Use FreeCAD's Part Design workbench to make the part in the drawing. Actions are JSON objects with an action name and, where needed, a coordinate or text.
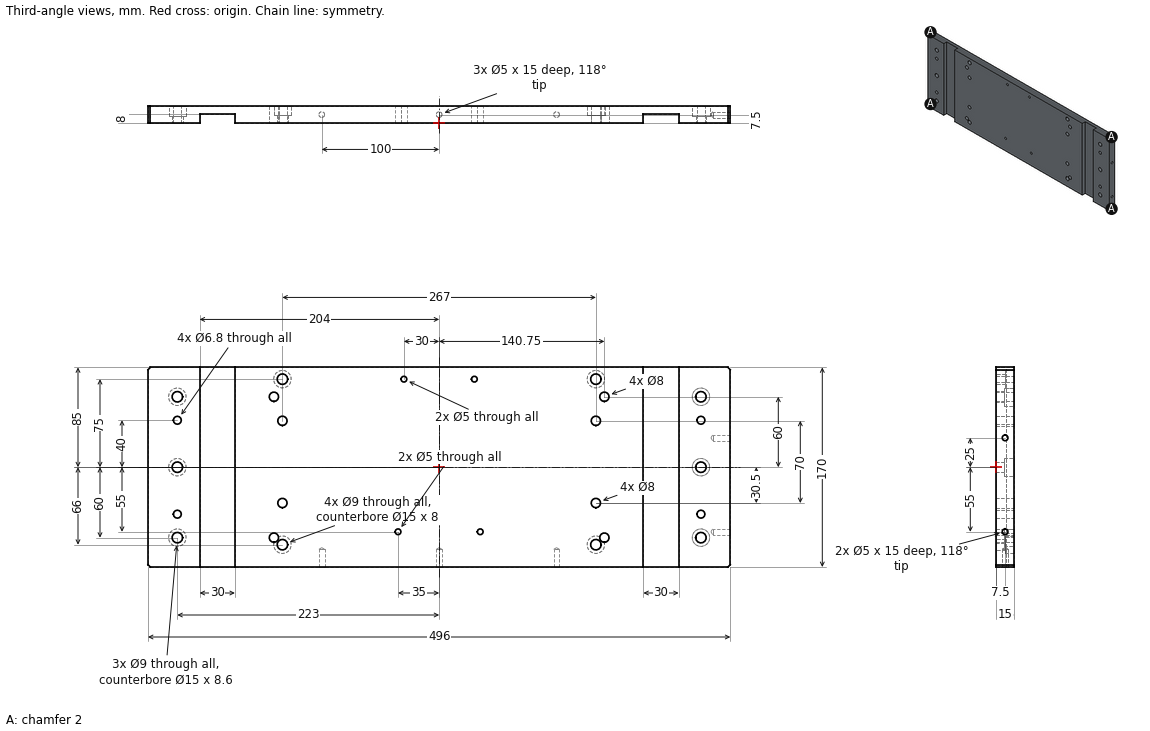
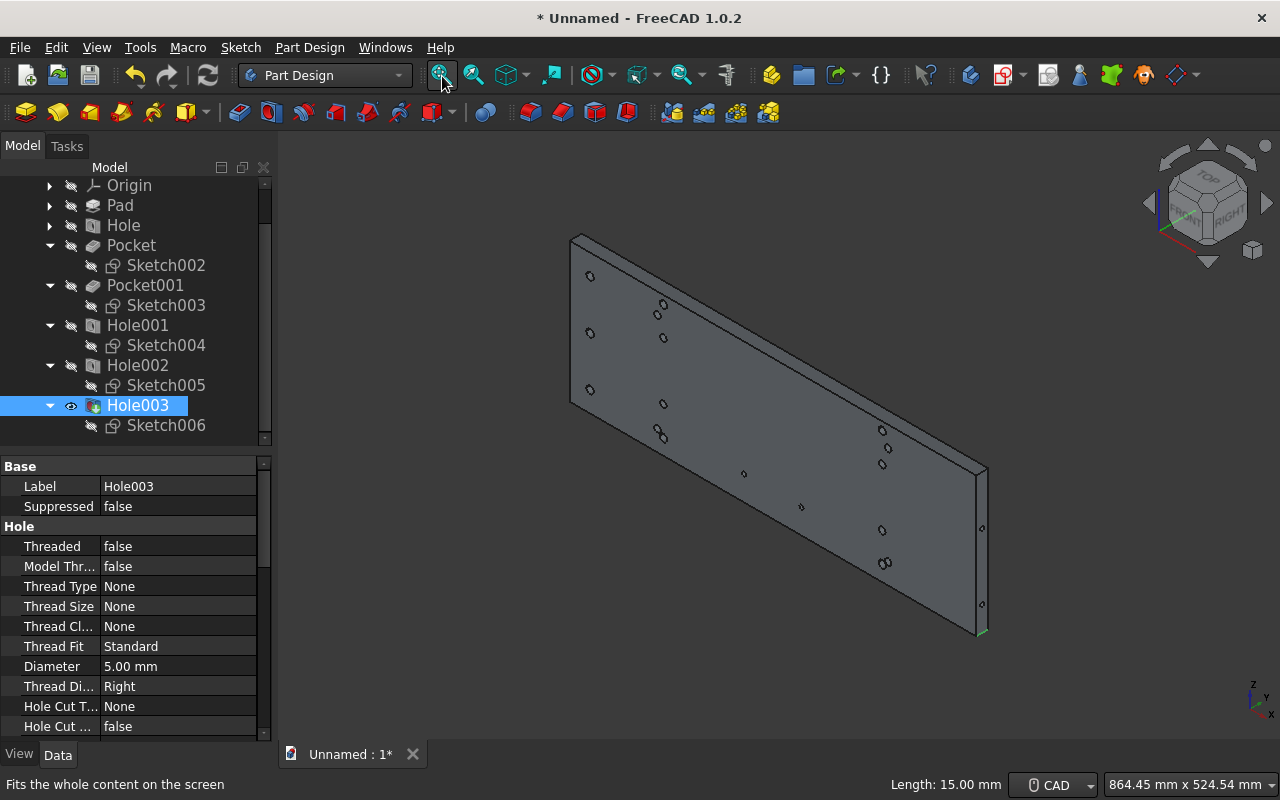
{"action": "left_click", "coordinate": [982, 471], "text": "ctrl"}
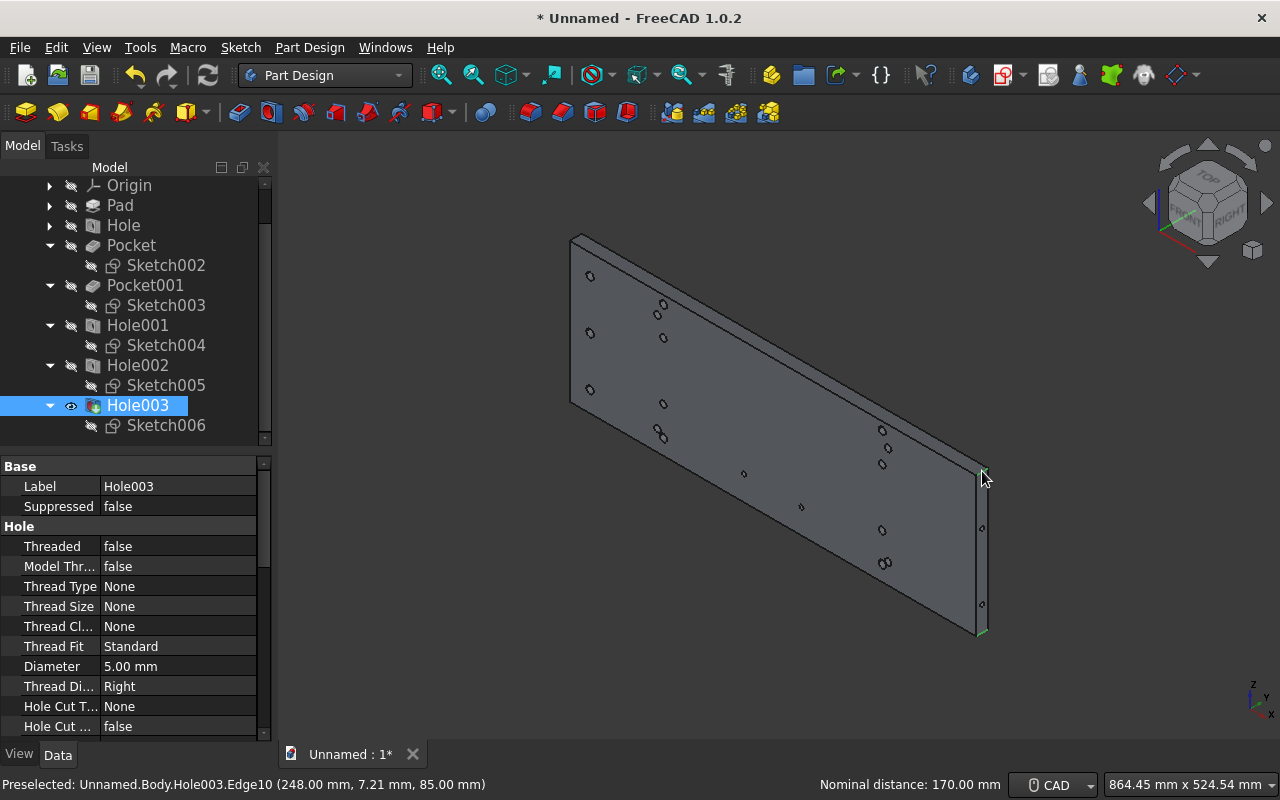
{"action": "scroll", "coordinate": [576, 236], "scroll_direction": "up", "scroll_amount": 5}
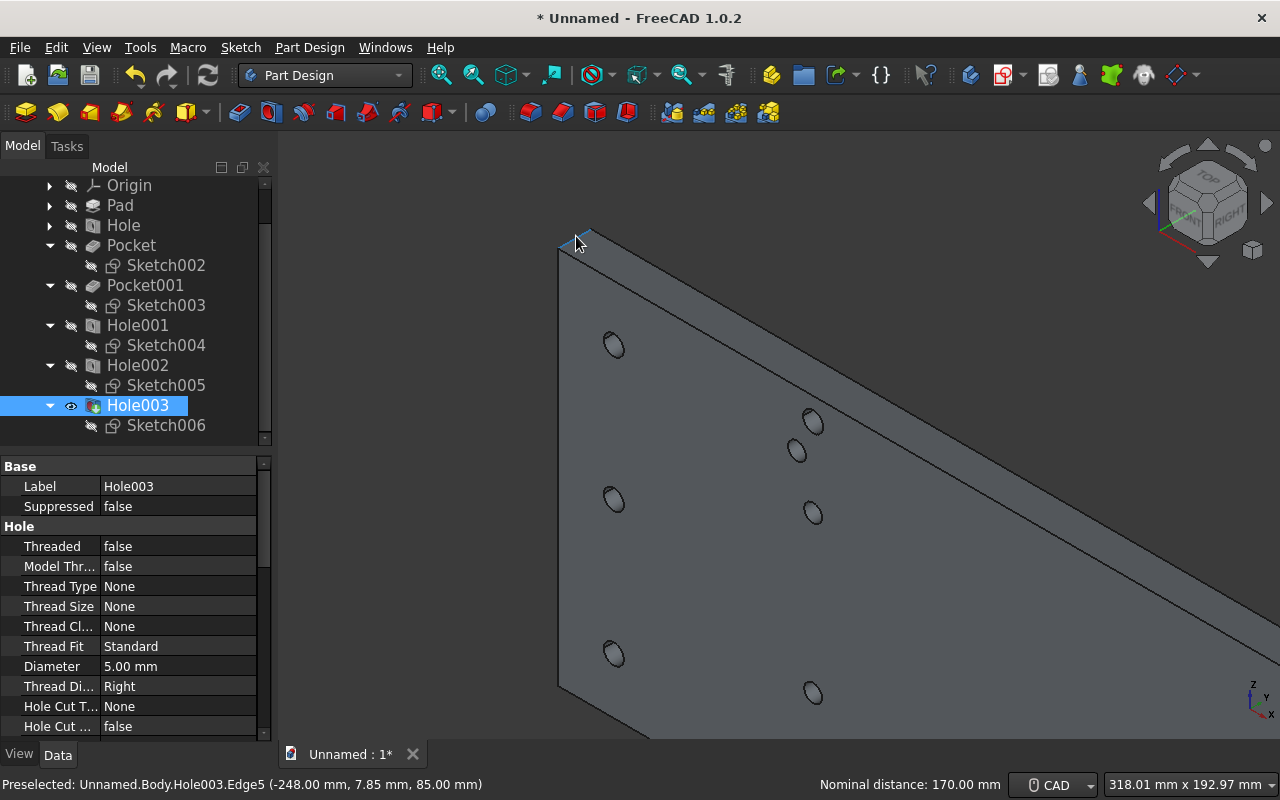
{"action": "left_click", "coordinate": [442, 76]}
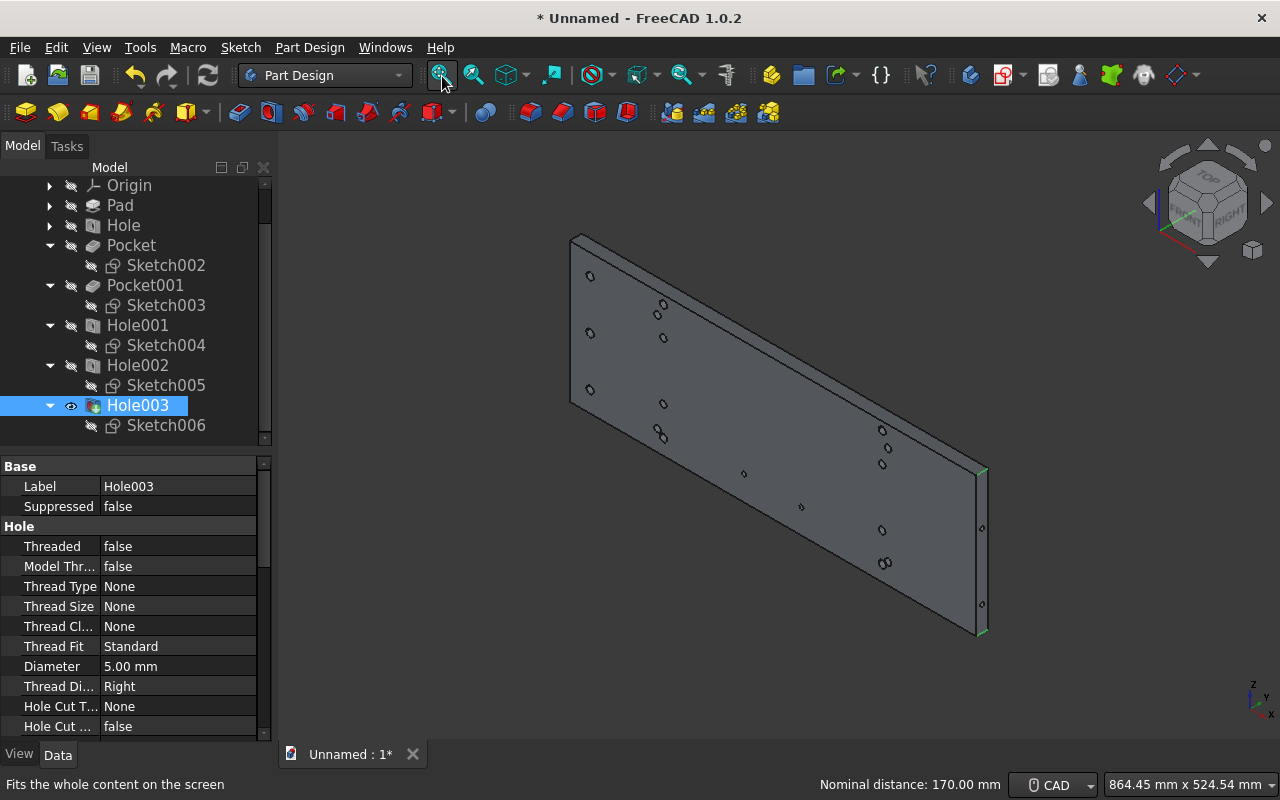
{"action": "key", "text": "2"}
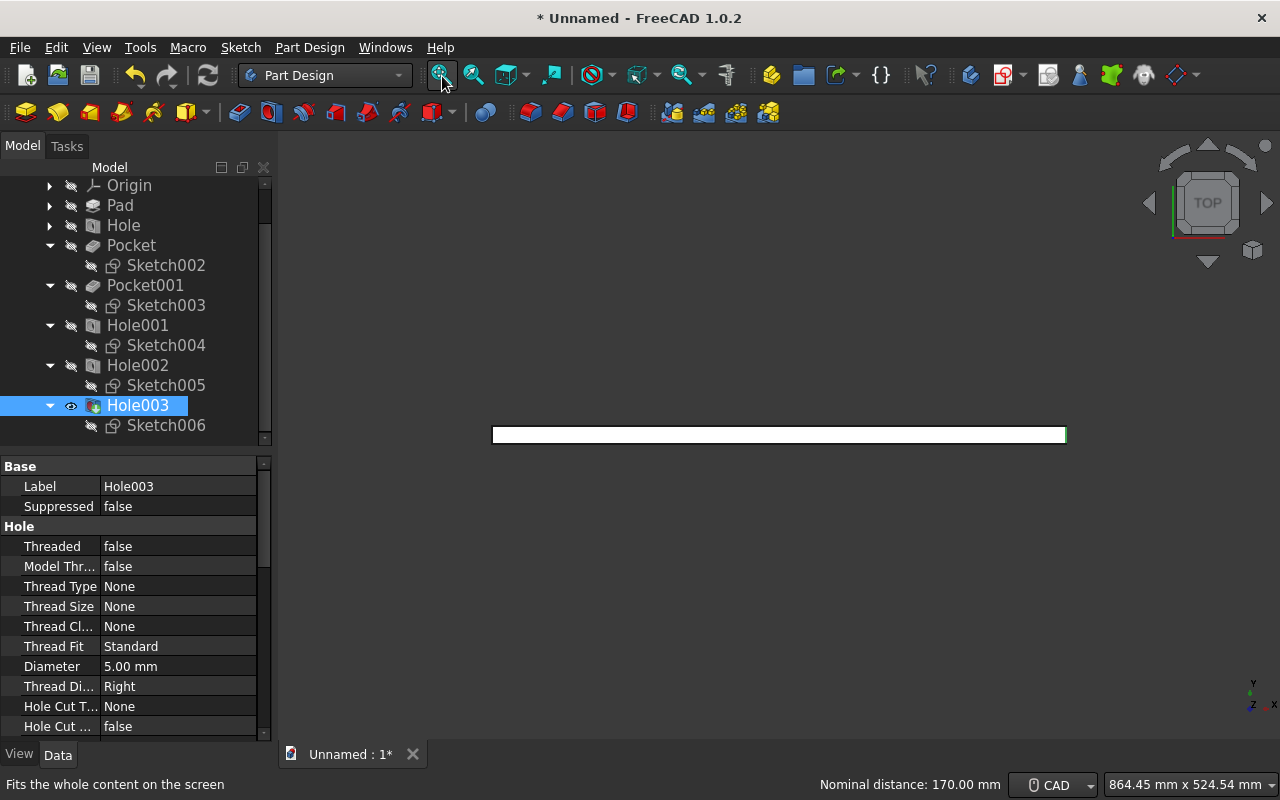
{"action": "left_click", "coordinate": [492, 434], "text": "ctrl"}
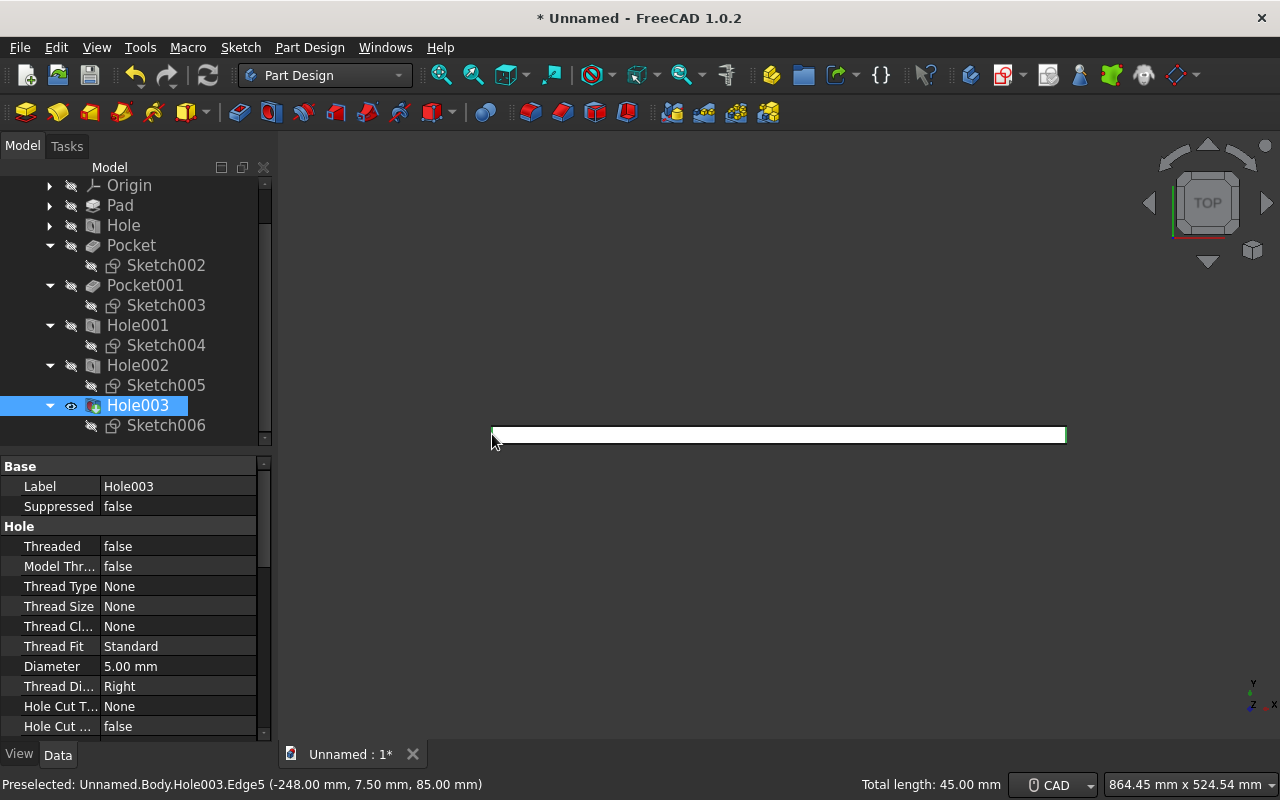
{"action": "scroll", "coordinate": [492, 434], "scroll_direction": "up", "scroll_amount": 5}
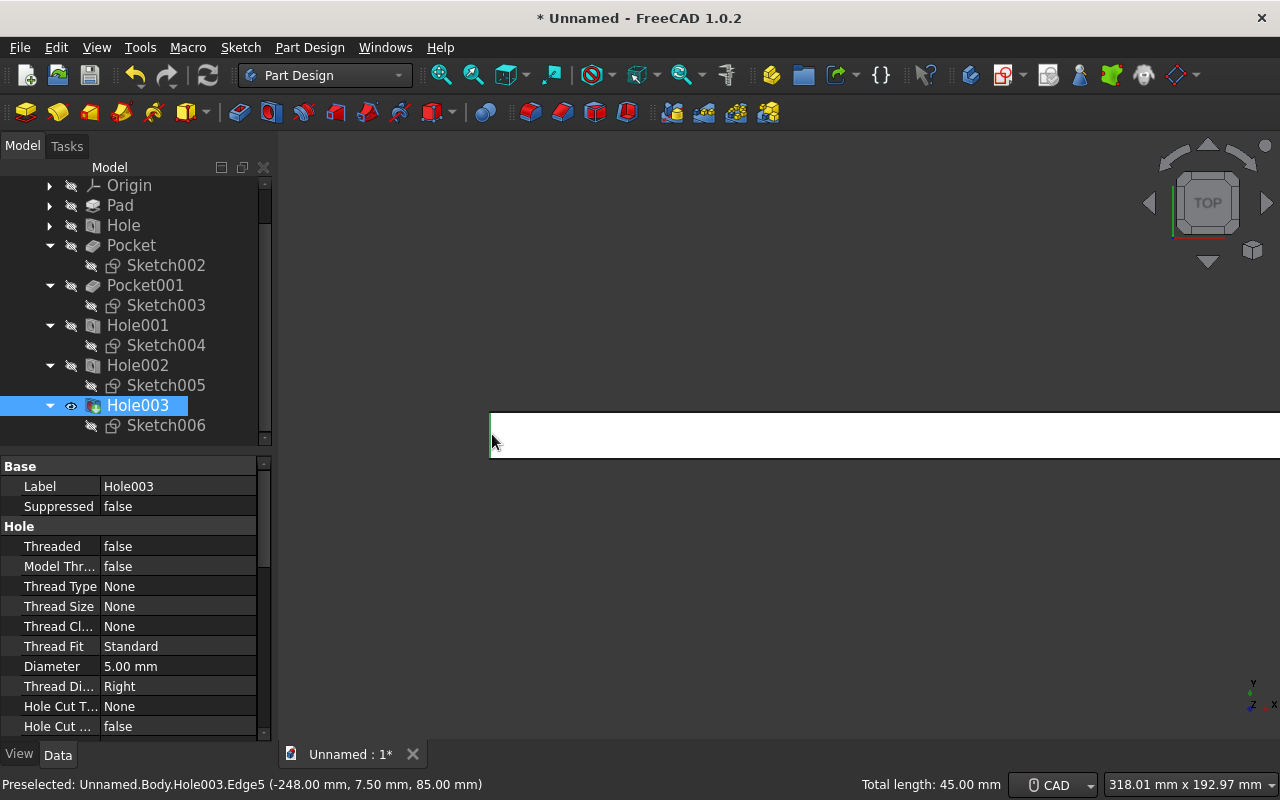
{"action": "left_click", "coordinate": [442, 76]}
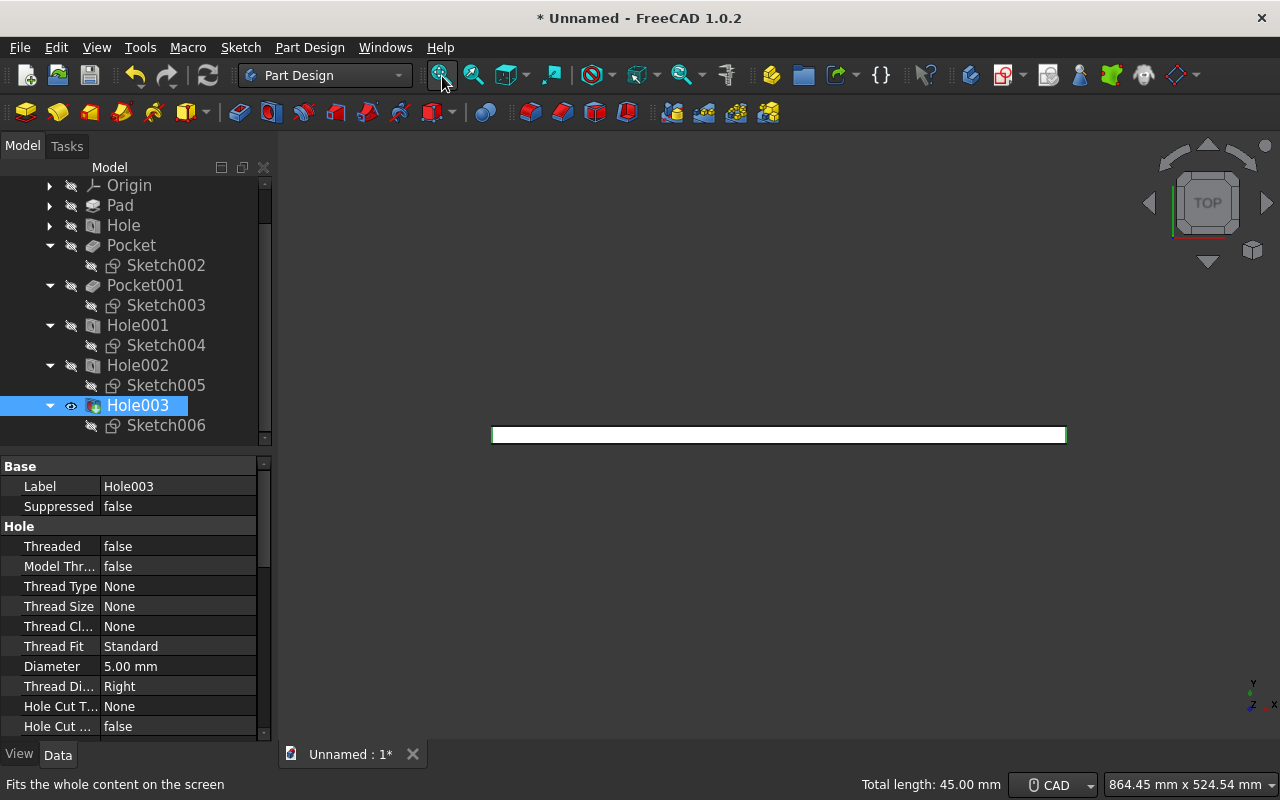
{"action": "key", "text": "1"}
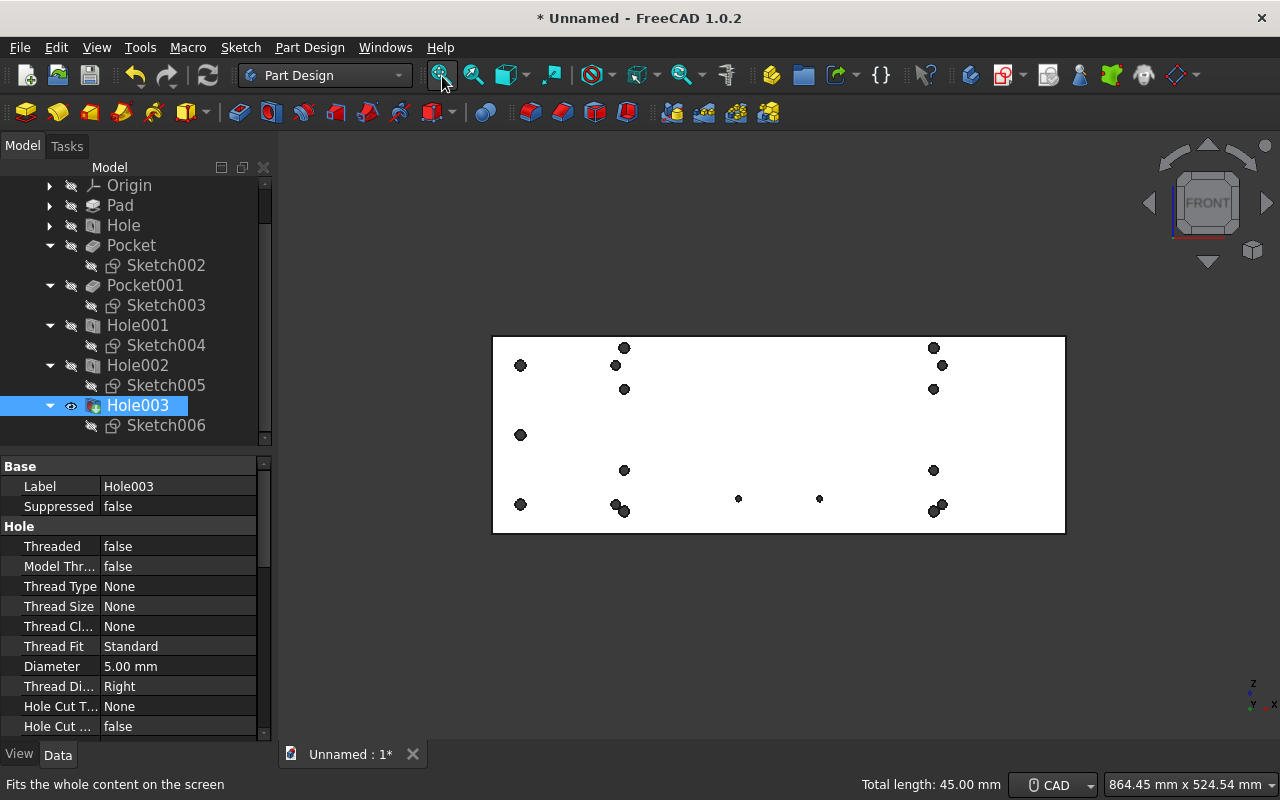
{"action": "scroll", "coordinate": [492, 533], "scroll_direction": "up", "scroll_amount": 5}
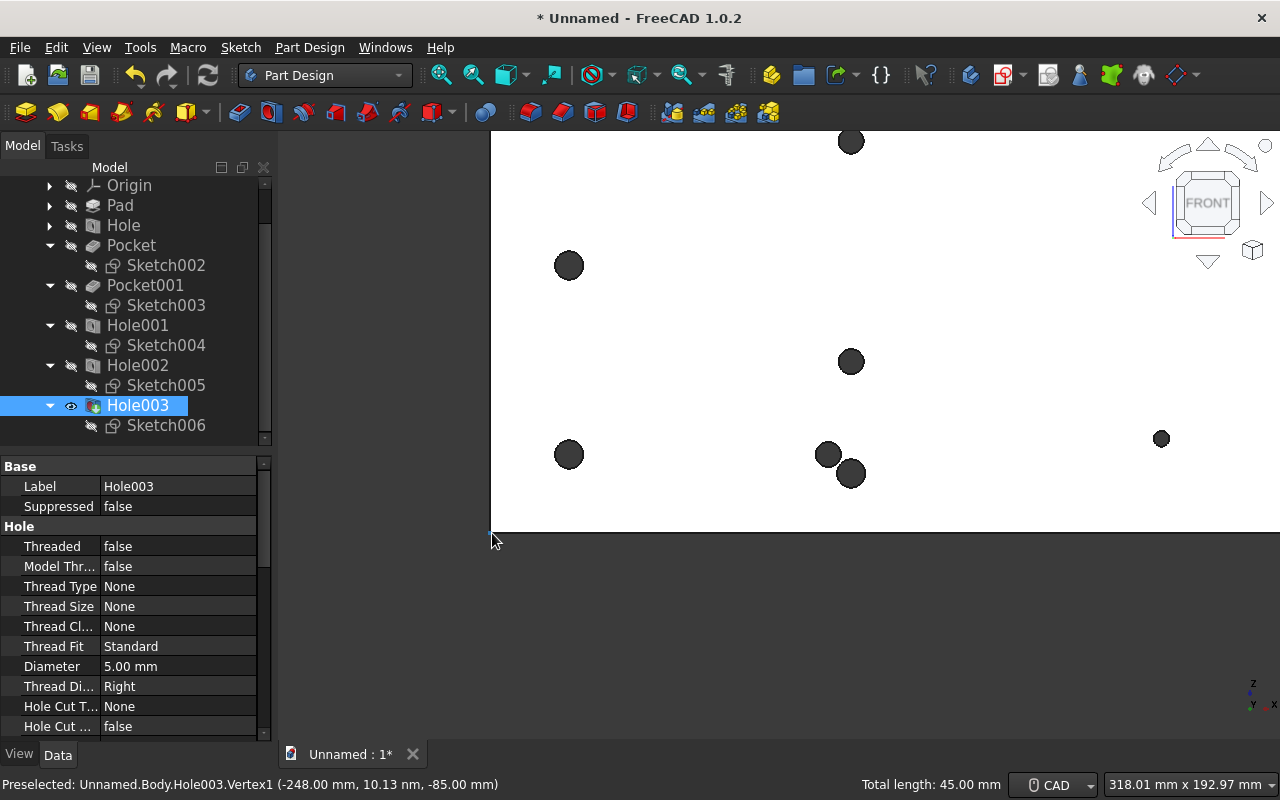
{"action": "left_click", "coordinate": [442, 76]}